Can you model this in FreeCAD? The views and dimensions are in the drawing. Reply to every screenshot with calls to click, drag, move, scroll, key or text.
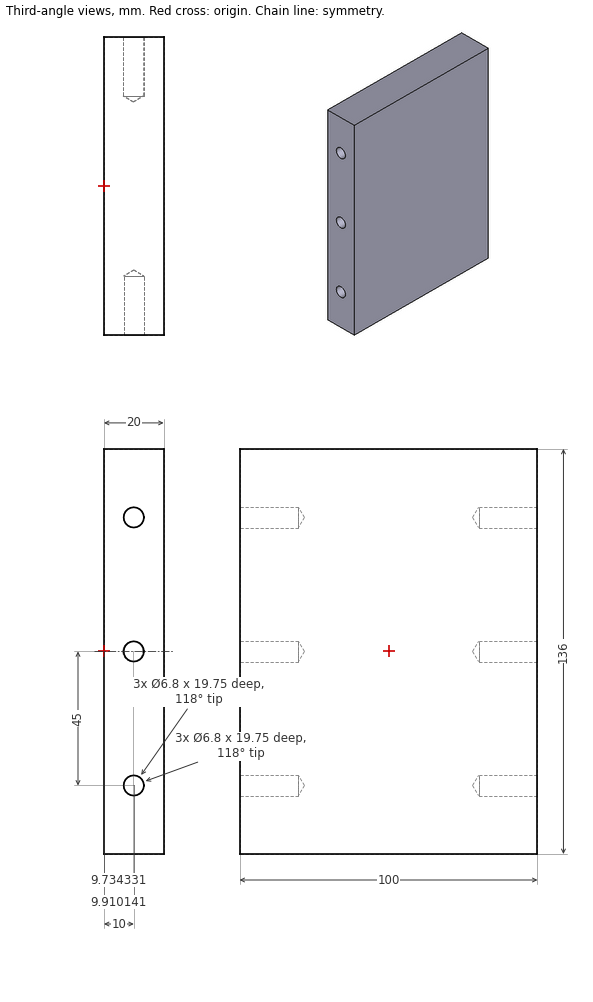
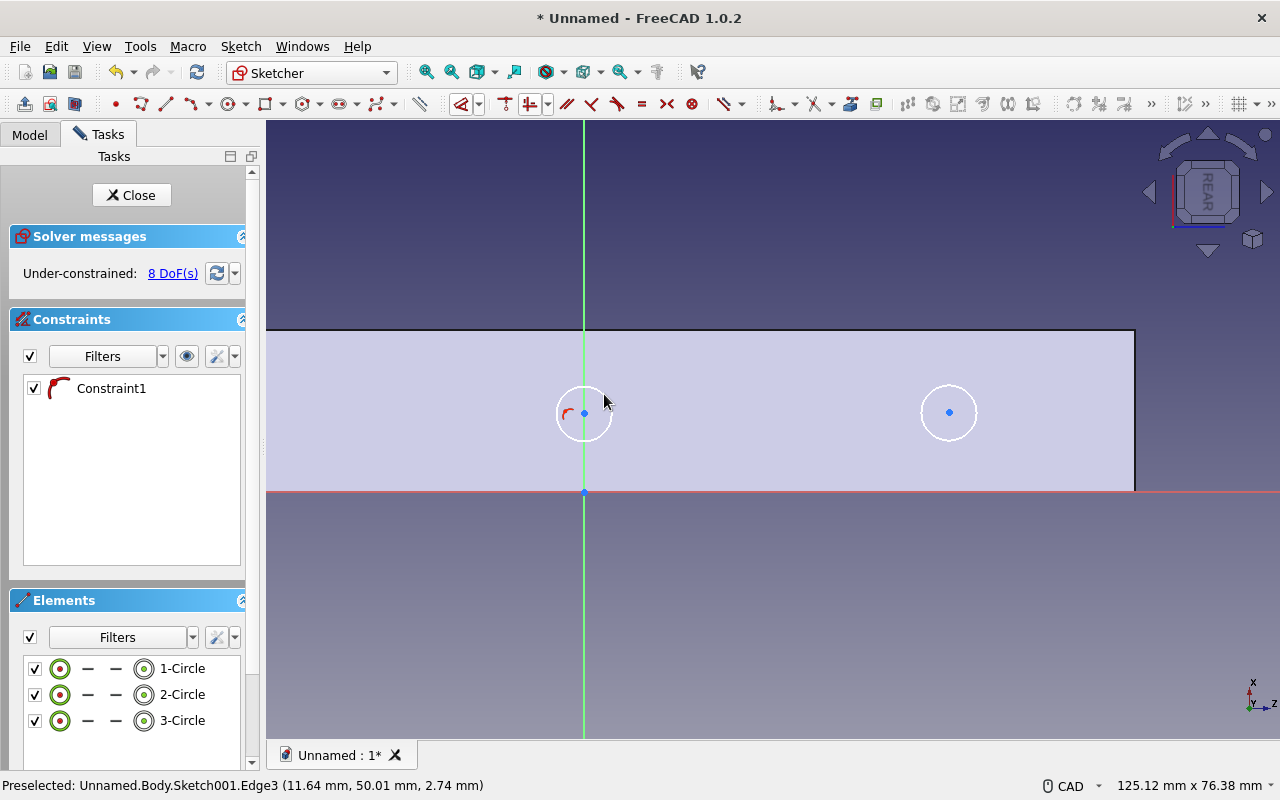
scroll(949, 412, down, 2)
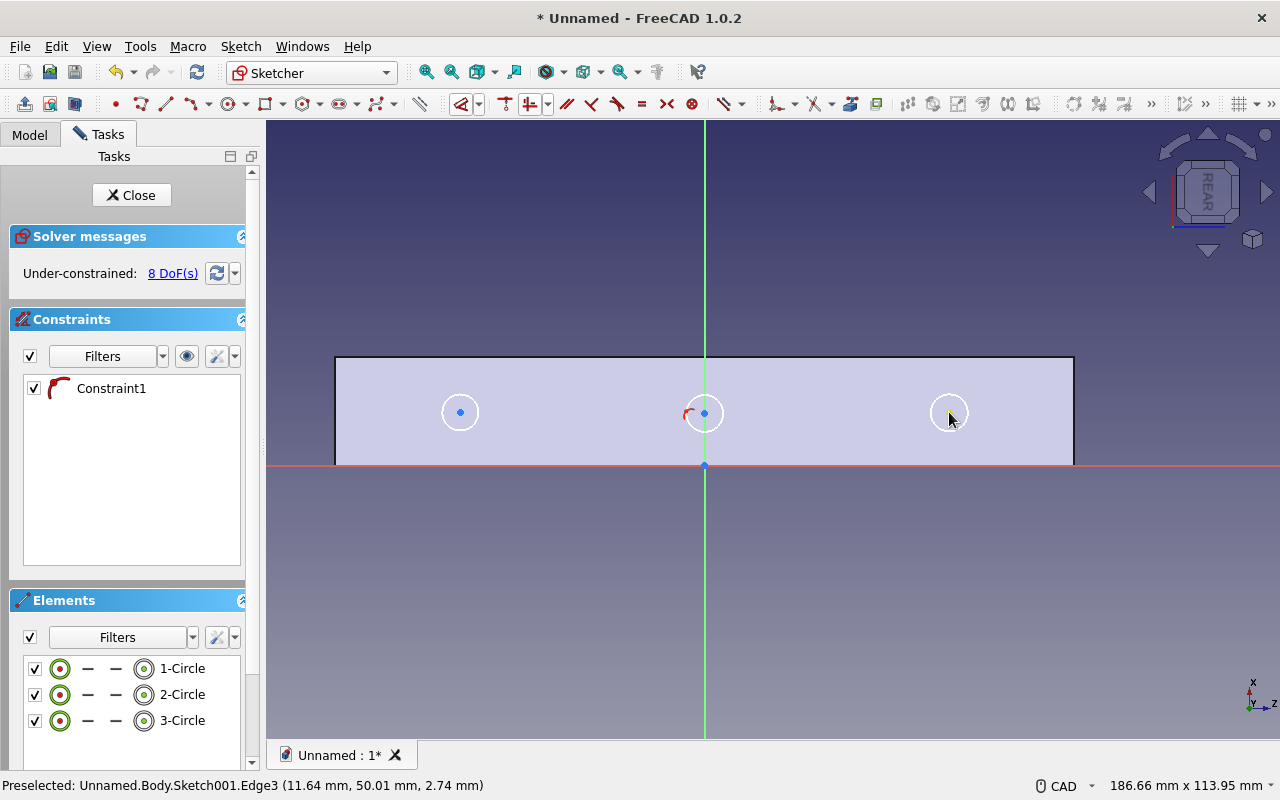
click(473, 400)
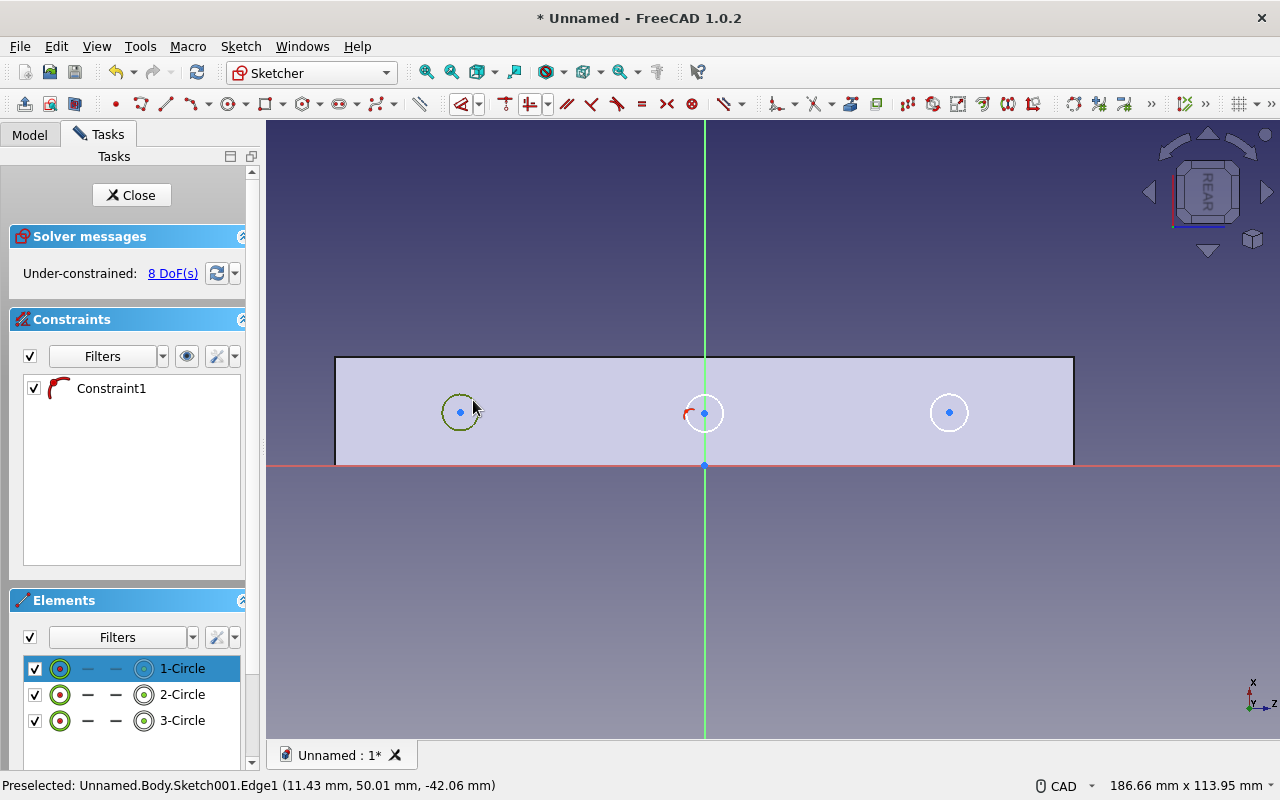
click(962, 400)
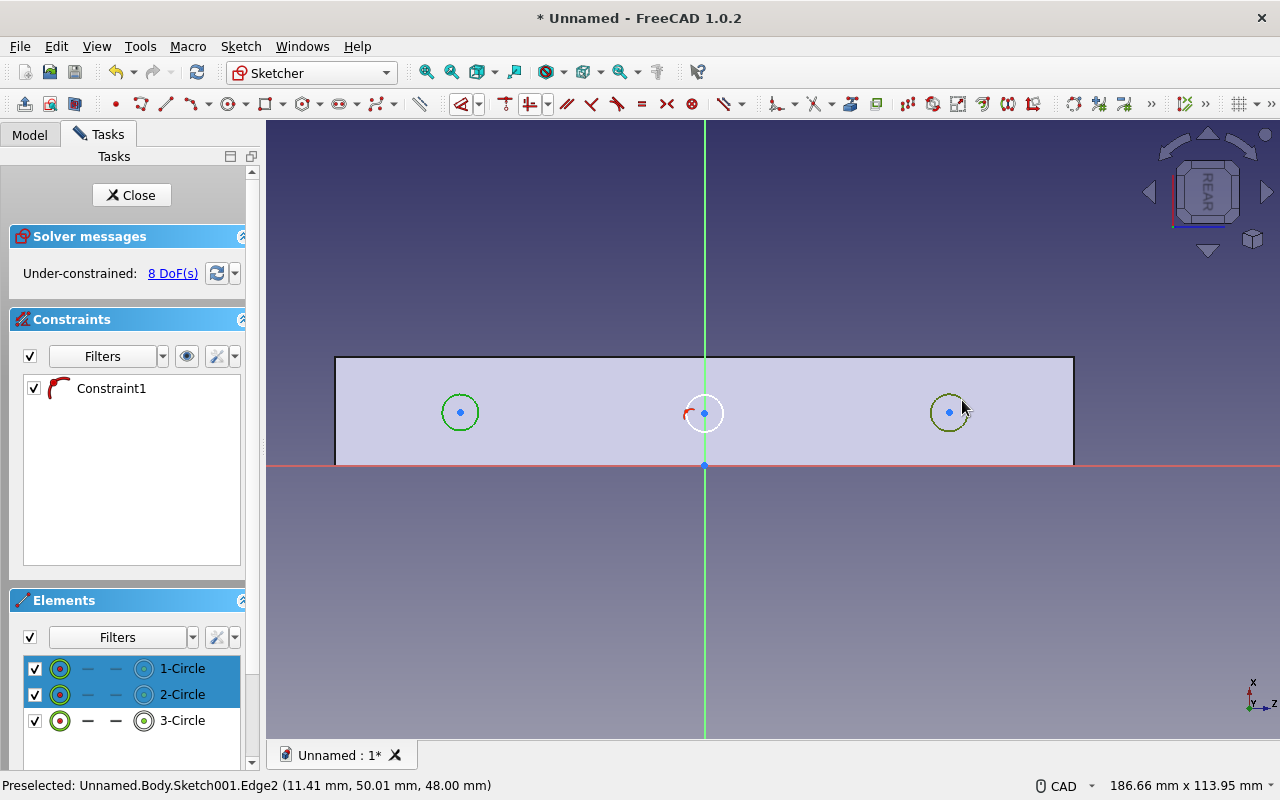
click(718, 400)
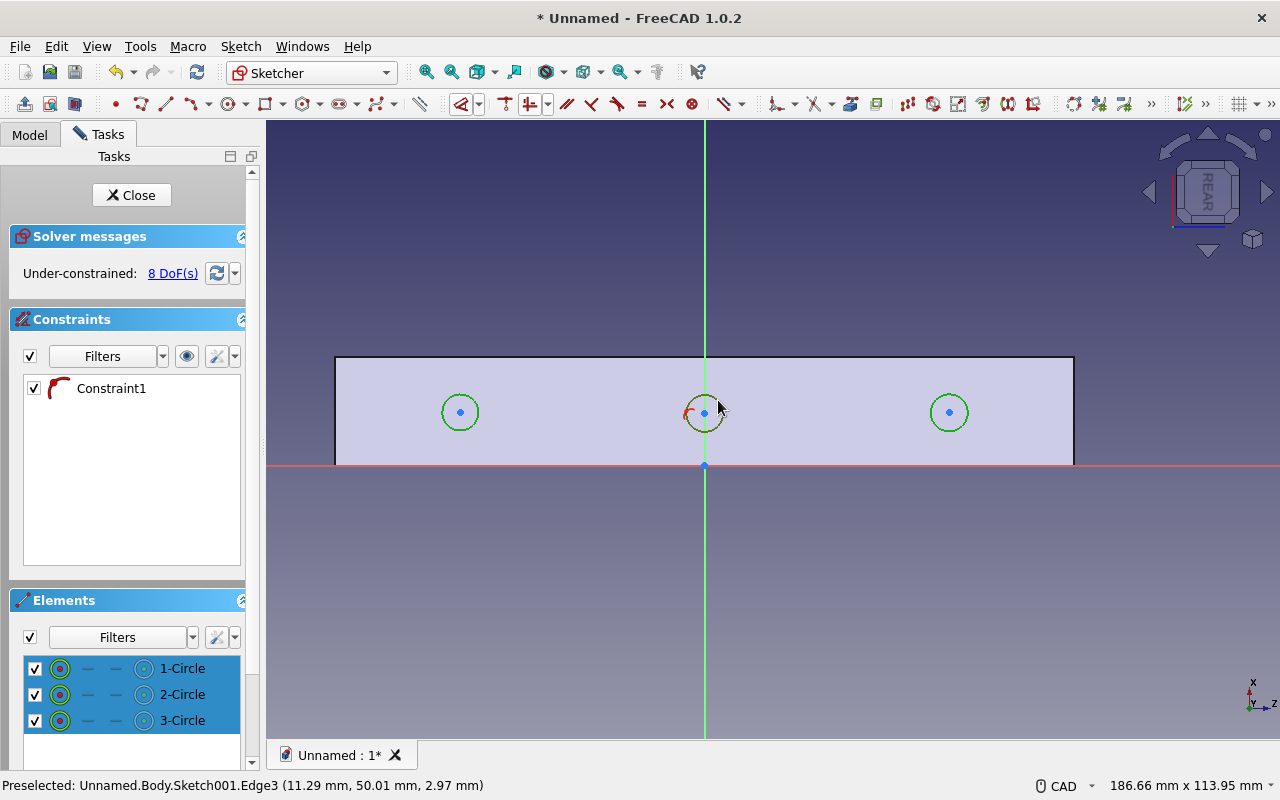
click(642, 104)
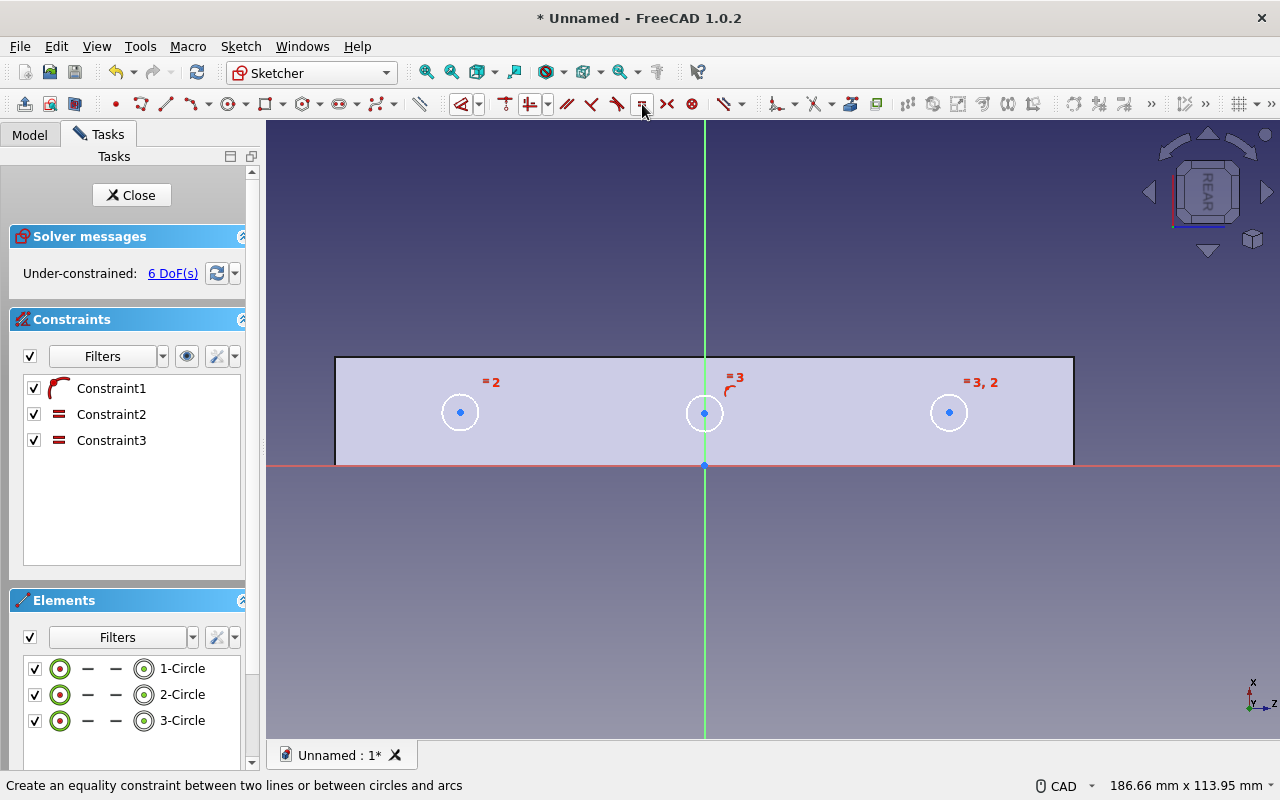
click(460, 412)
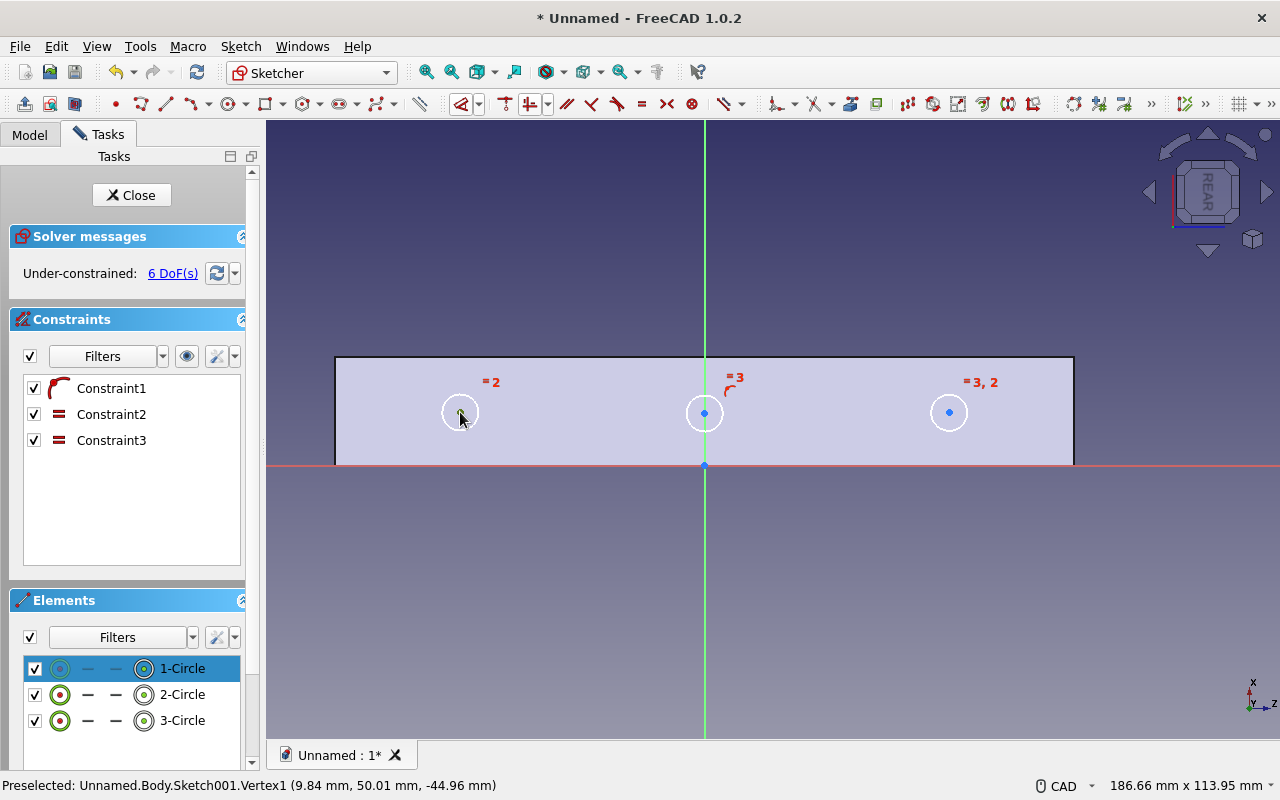
click(949, 413)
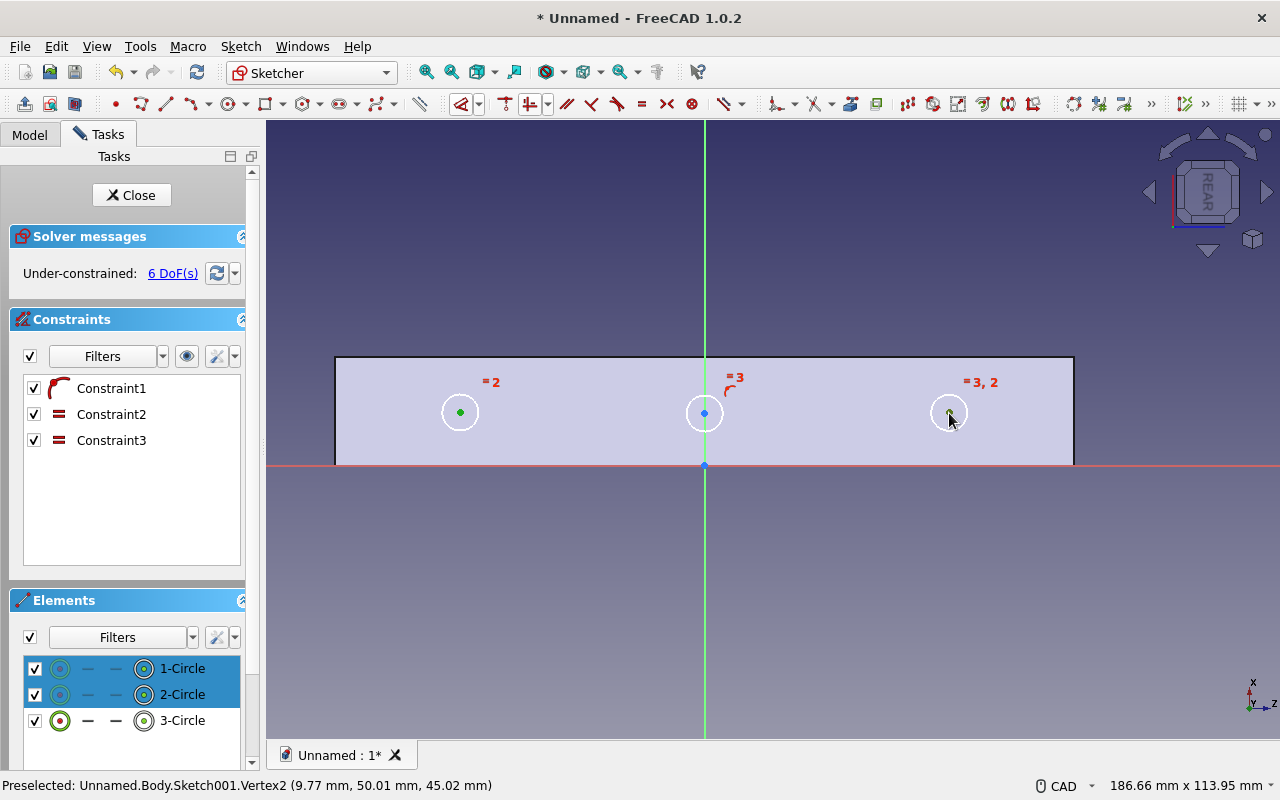
click(705, 671)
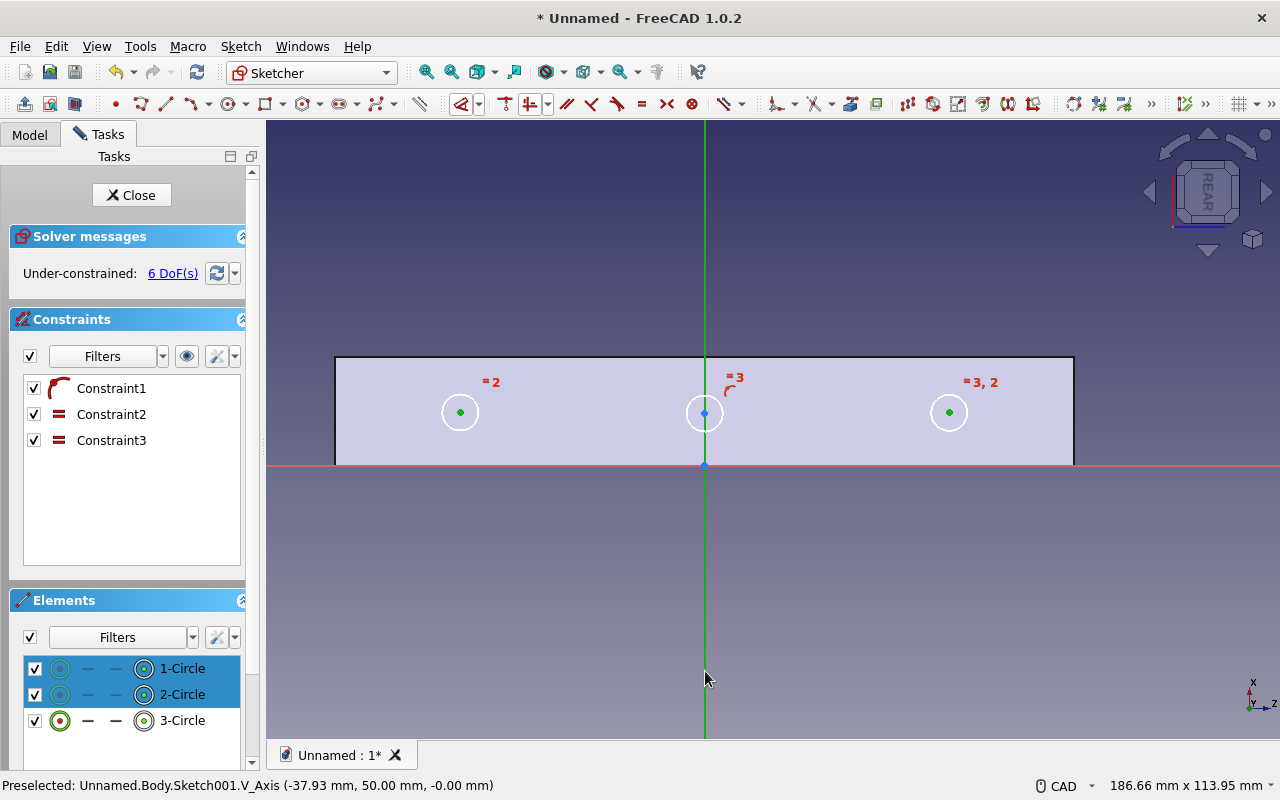
click(667, 104)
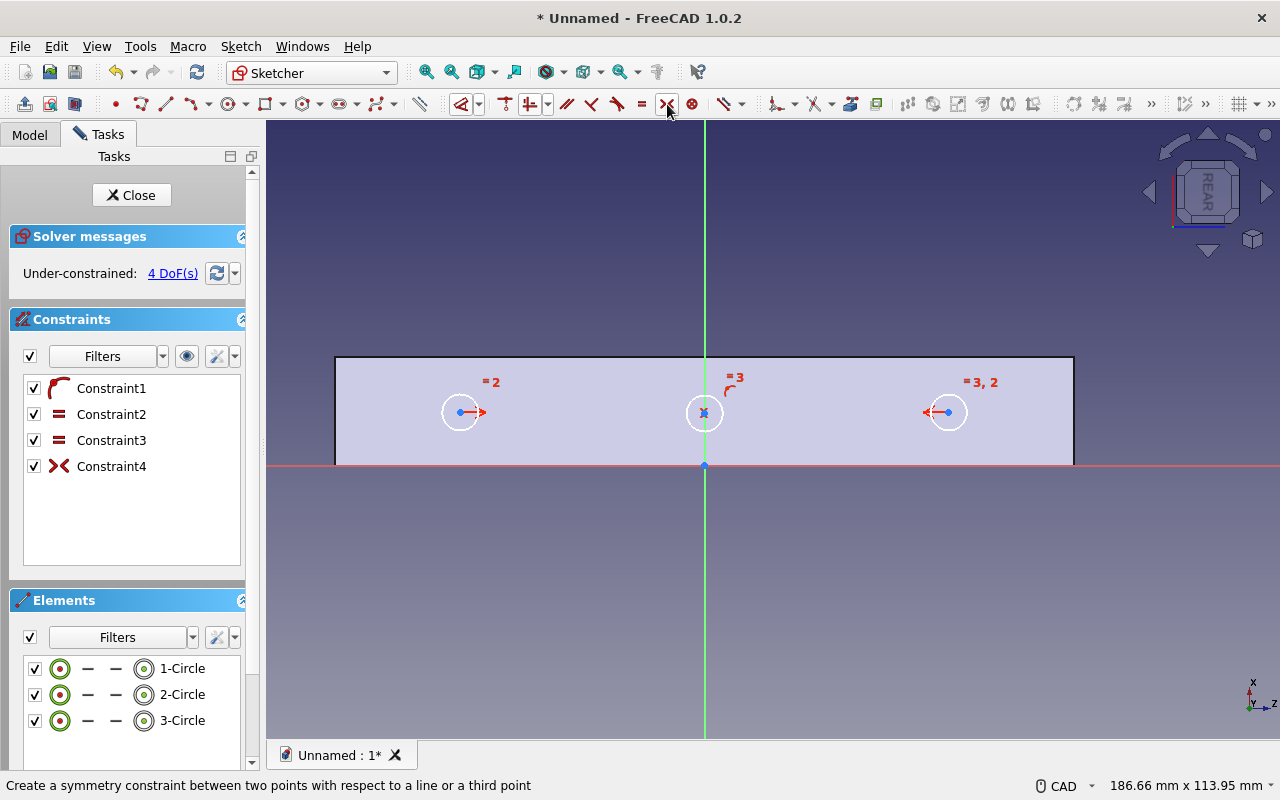
click(473, 400)